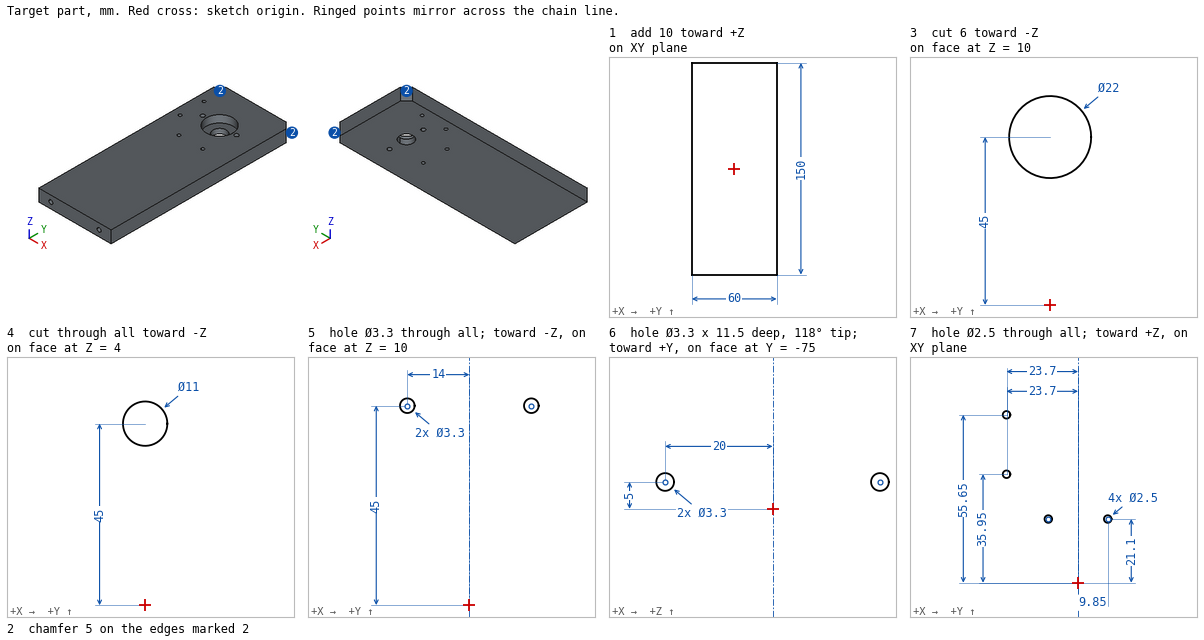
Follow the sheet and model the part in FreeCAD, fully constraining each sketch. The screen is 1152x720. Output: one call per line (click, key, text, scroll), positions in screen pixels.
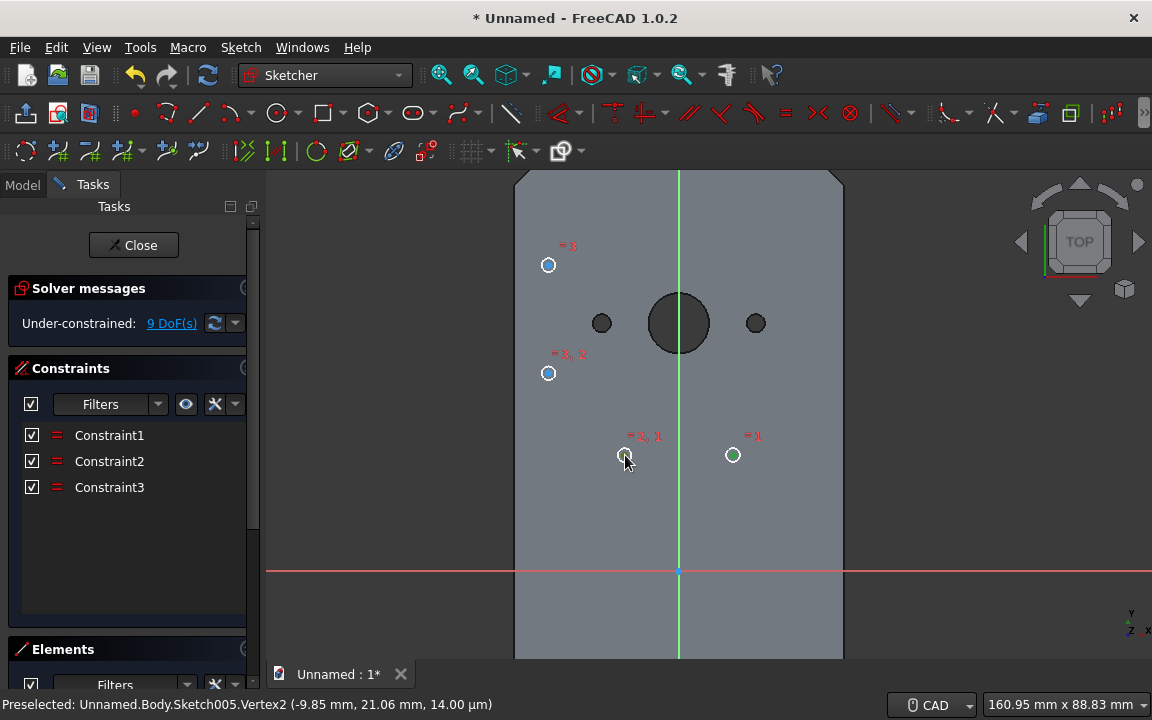
click(679, 538)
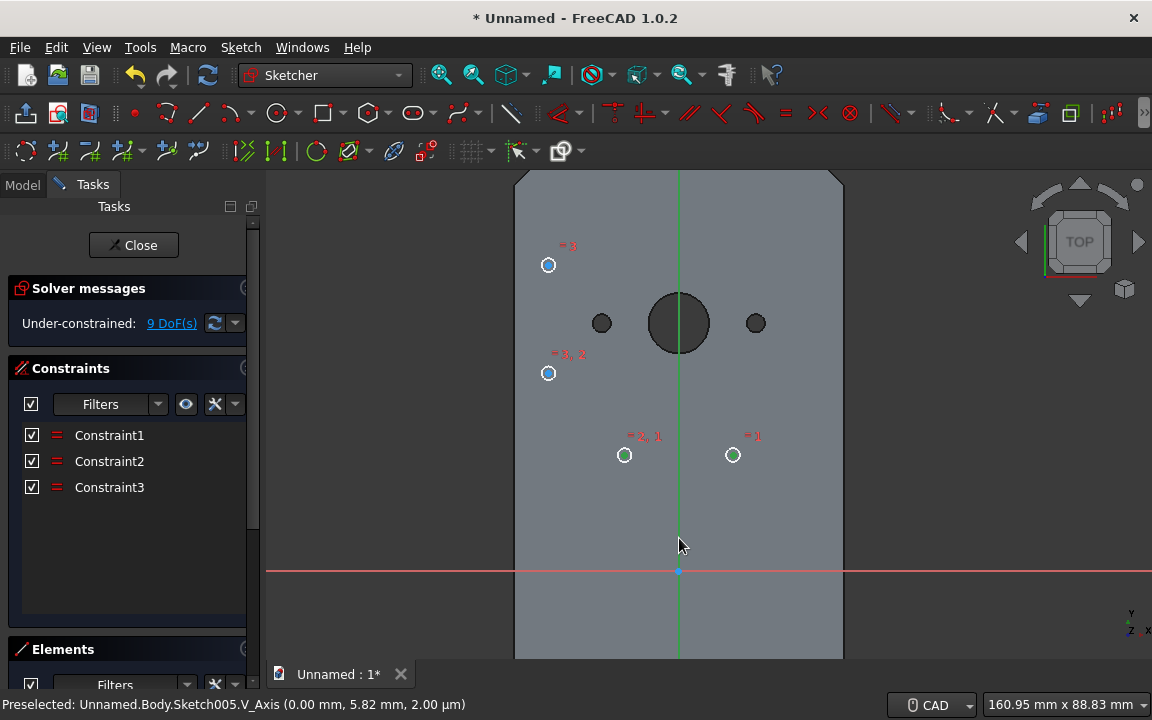
click(818, 114)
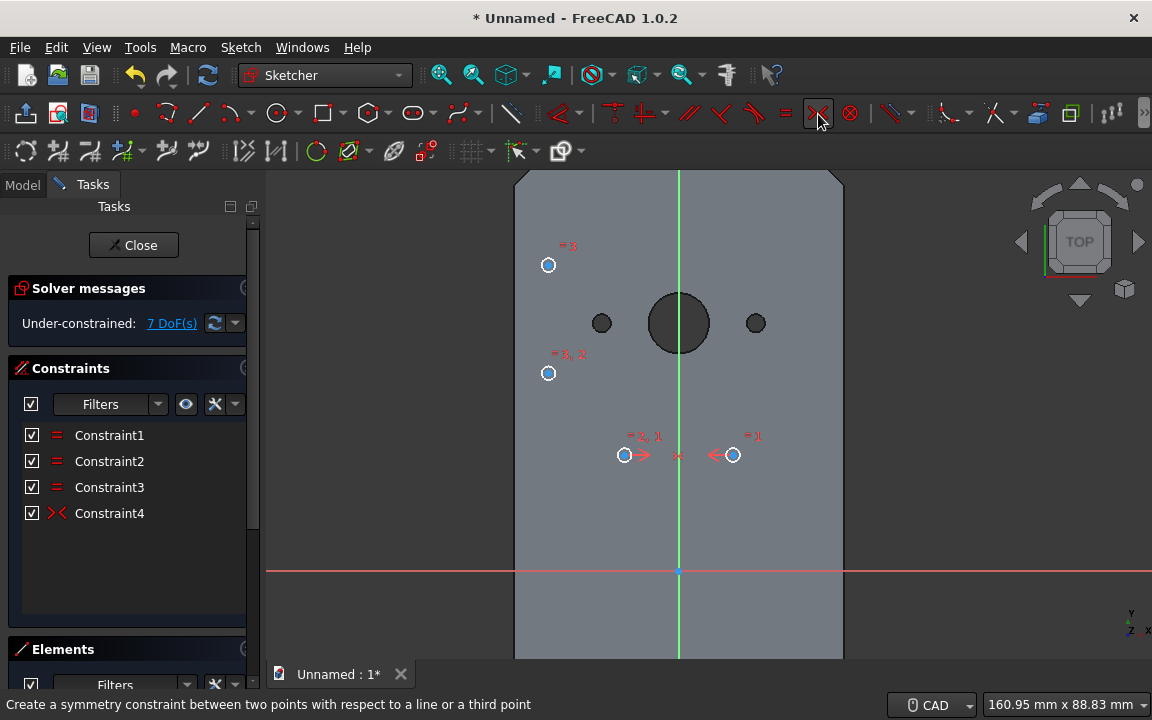
click(558, 114)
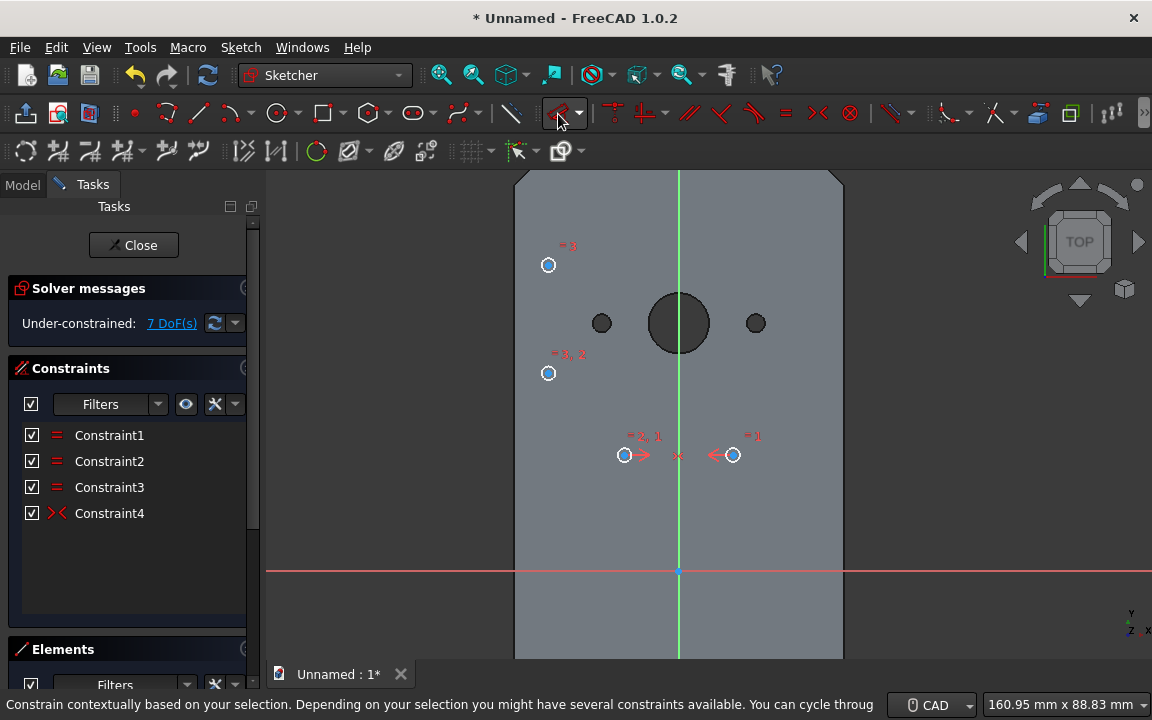
scroll(733, 448, up, 6)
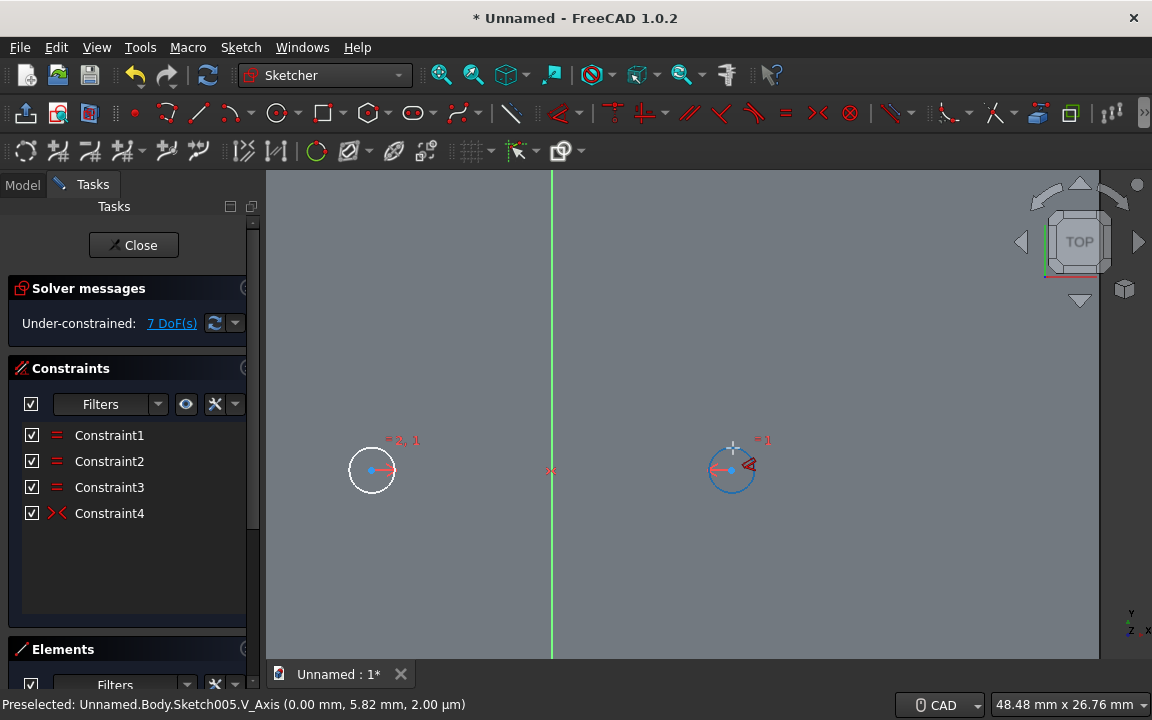
click(733, 448)
click(735, 416)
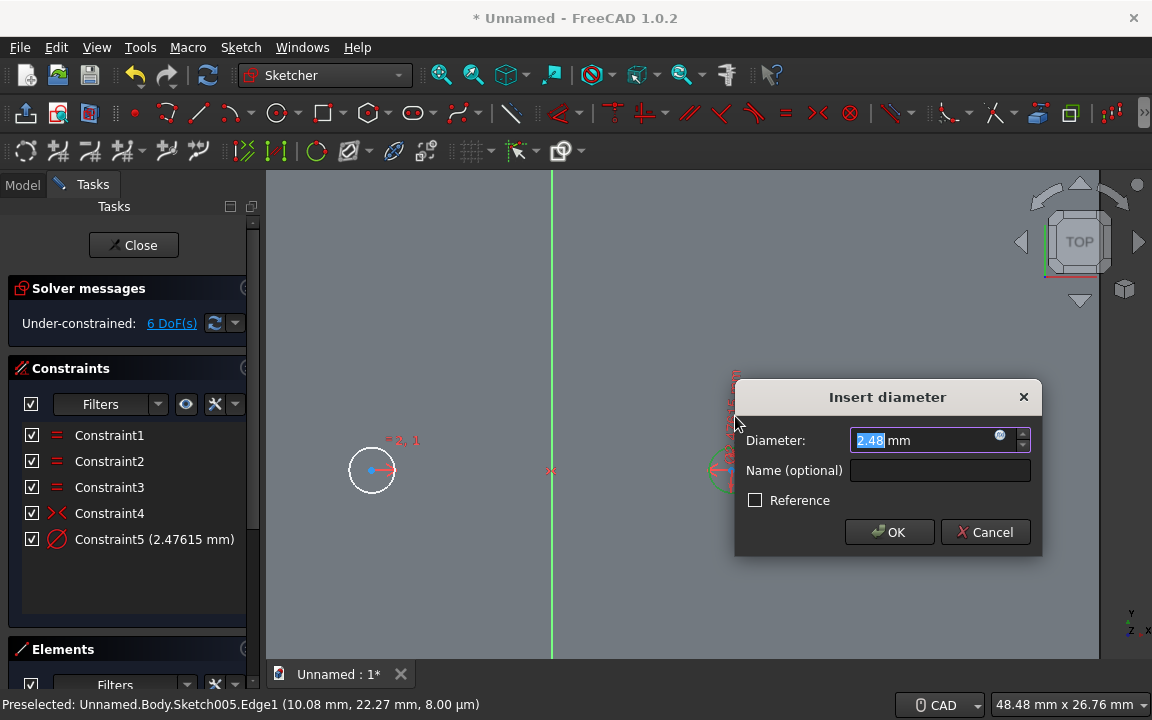
text(2.5)
key(Return)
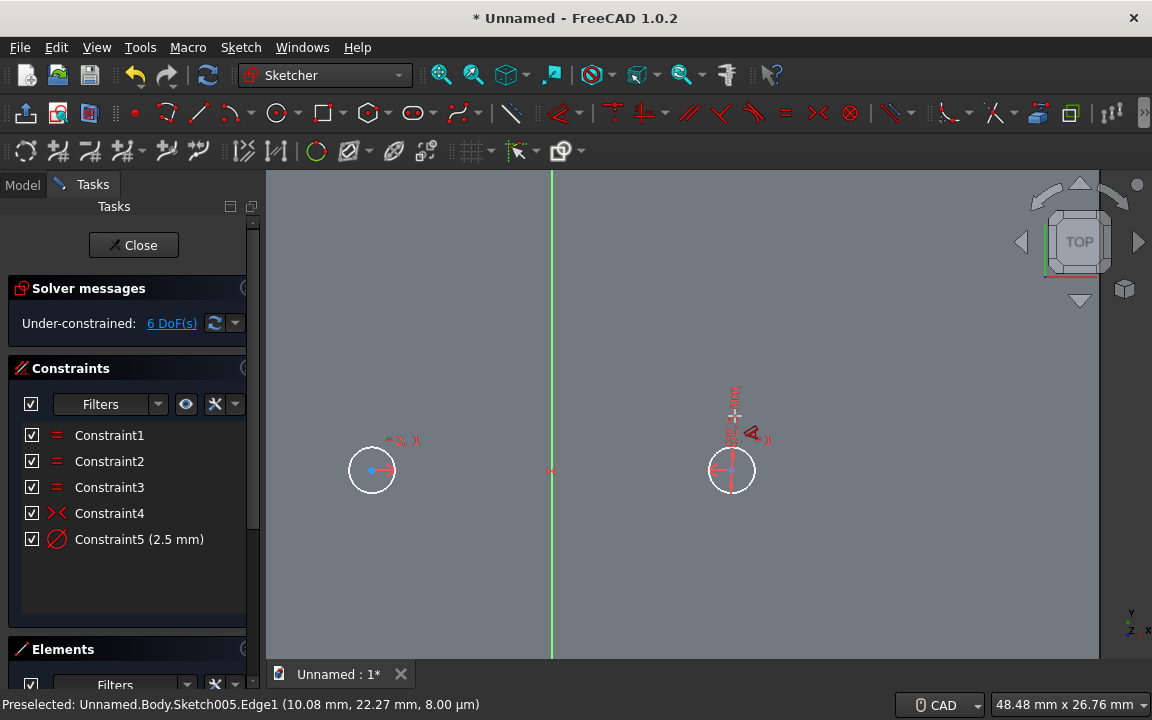
click(732, 470)
click(642, 436)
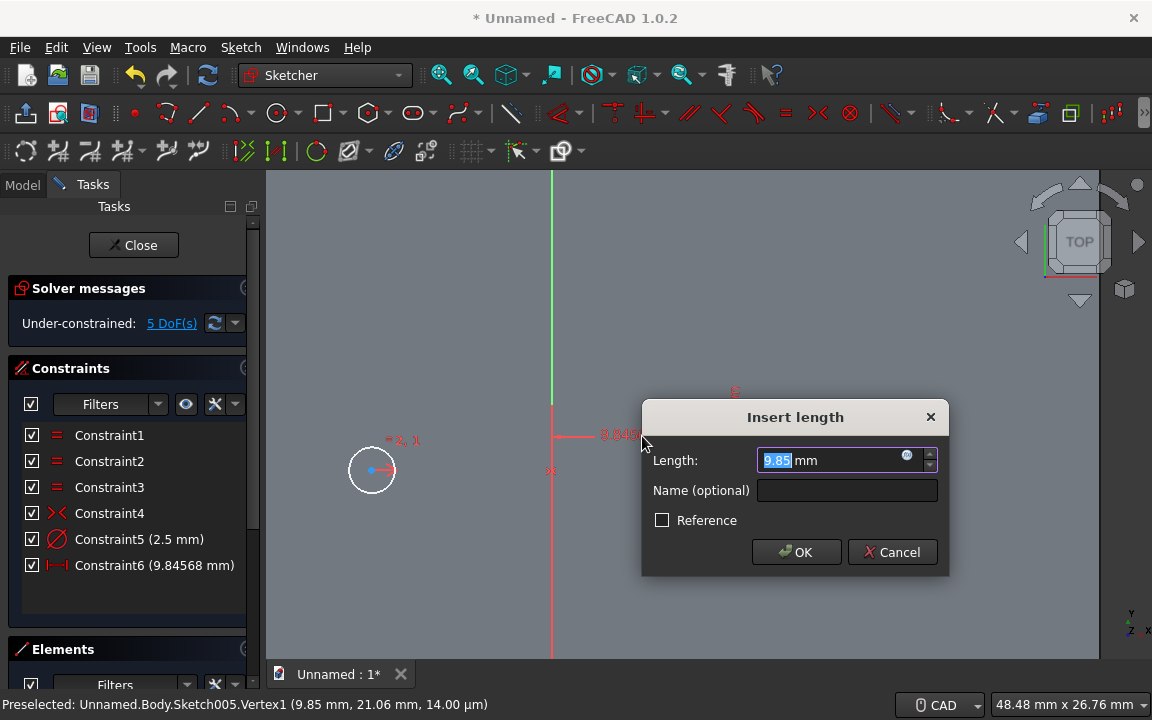
text(9.85)
key(Return)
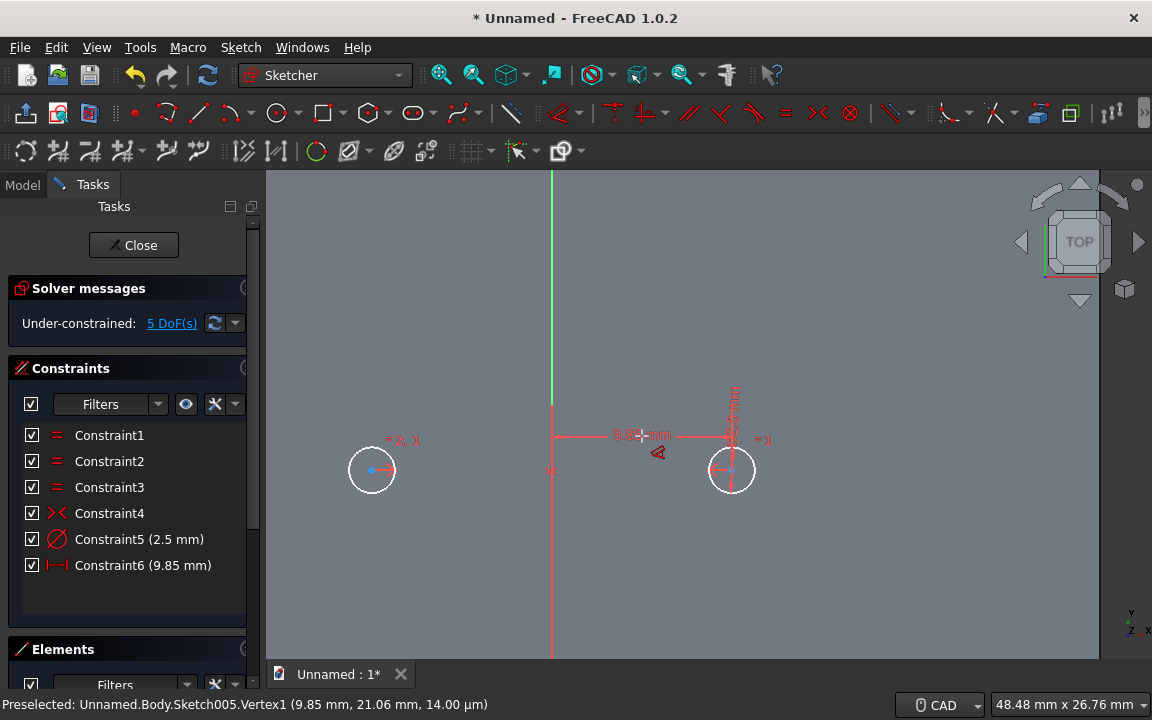
click(732, 470)
click(766, 551)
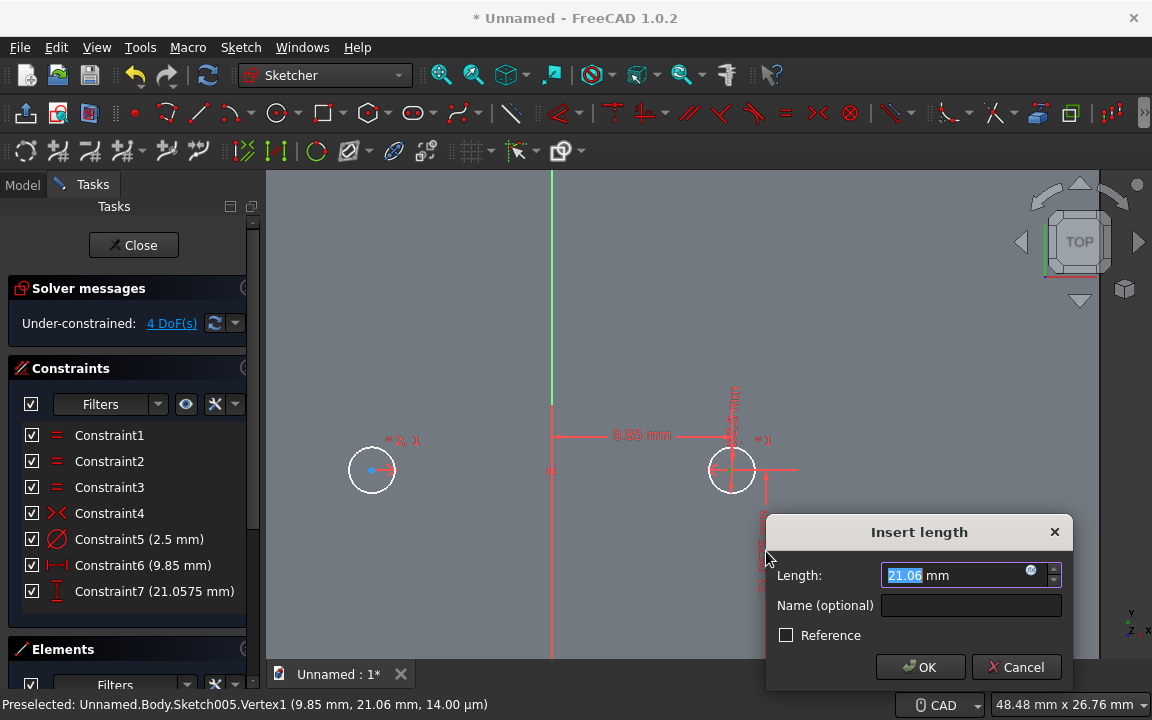
text(21.1)
key(Return)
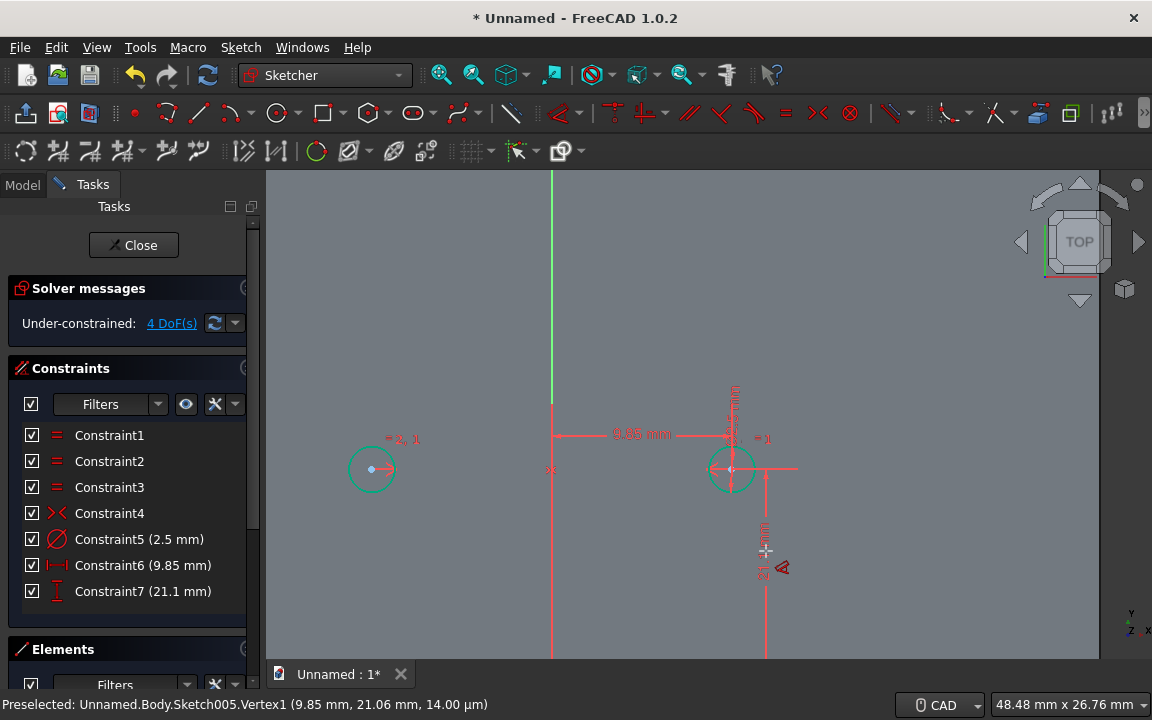
scroll(733, 449, down, 6)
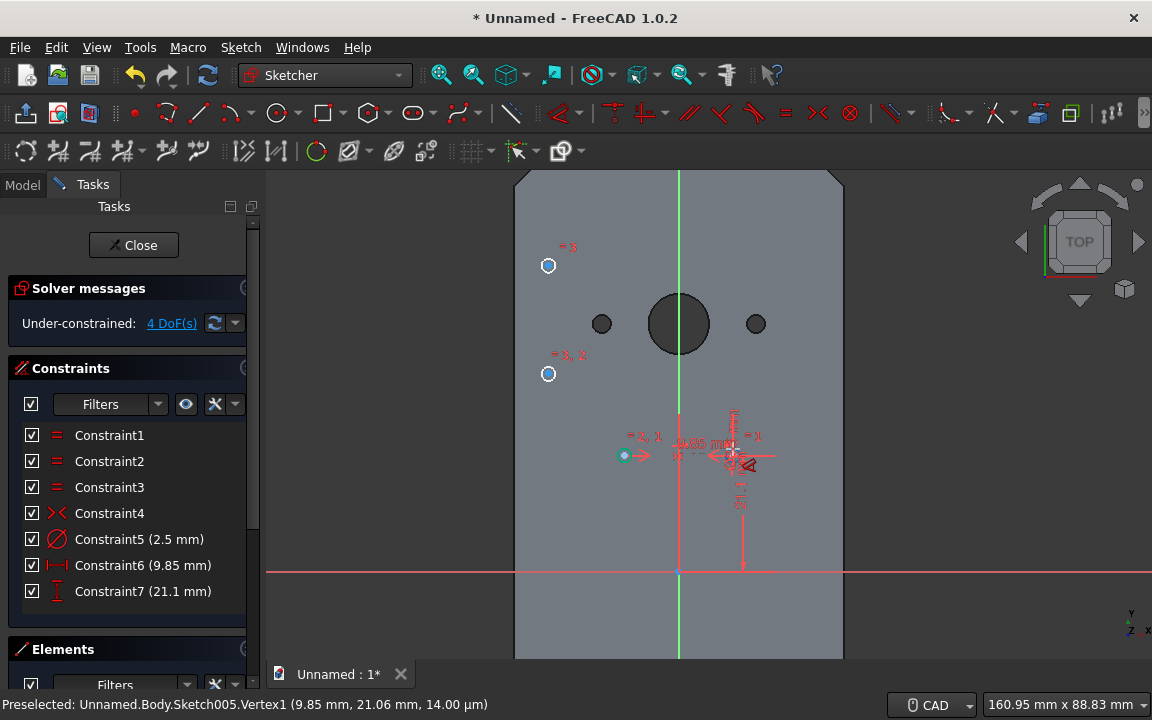
click(549, 374)
click(614, 606)